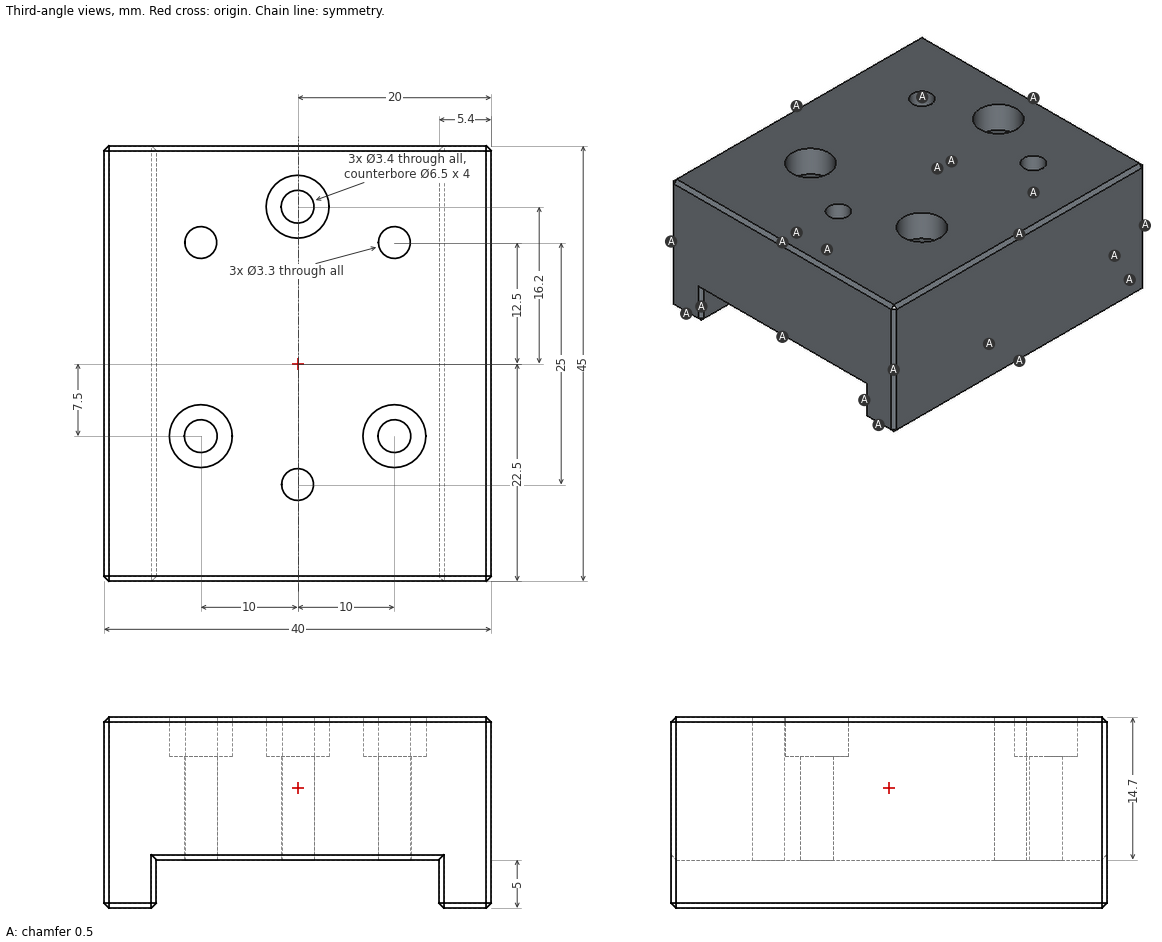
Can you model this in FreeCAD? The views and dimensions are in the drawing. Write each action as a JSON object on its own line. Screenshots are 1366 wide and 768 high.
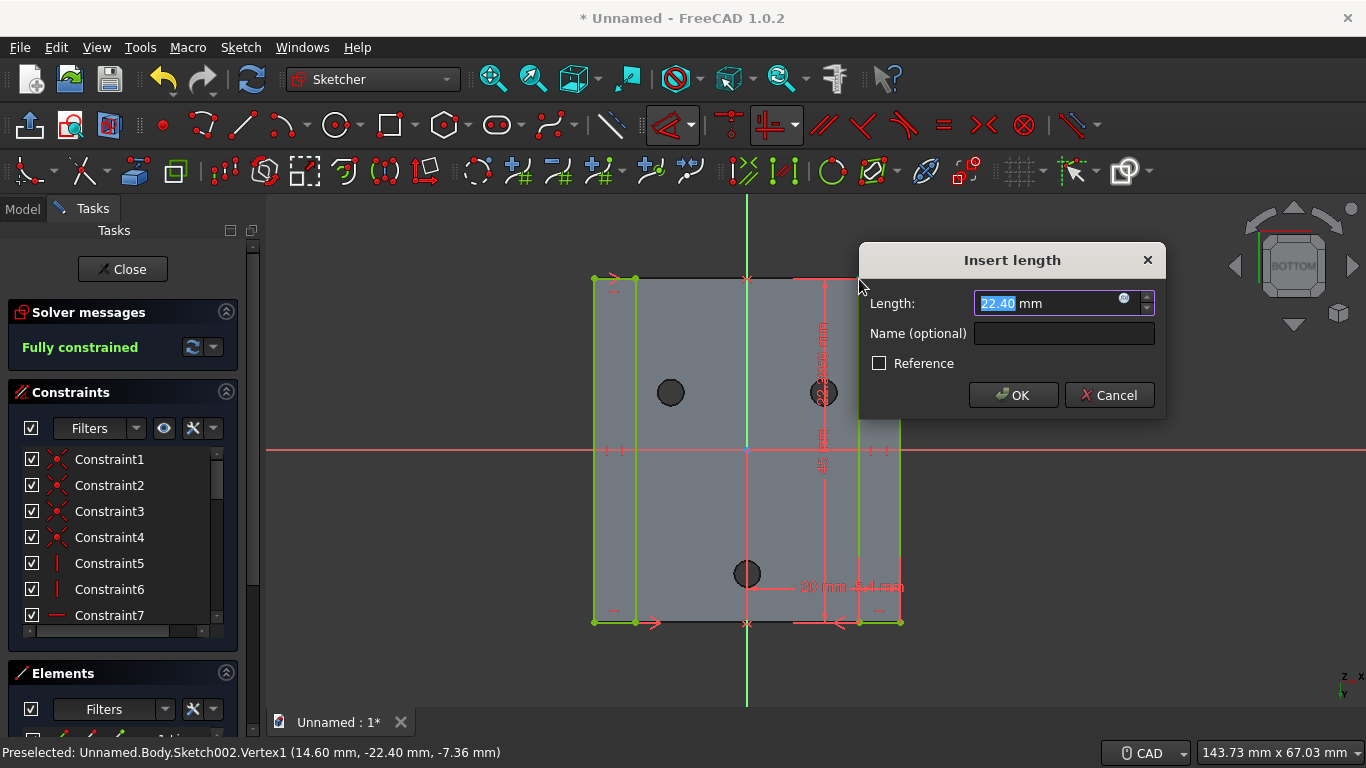
{"action": "type", "text": "22.5"}
{"action": "key", "text": "Return"}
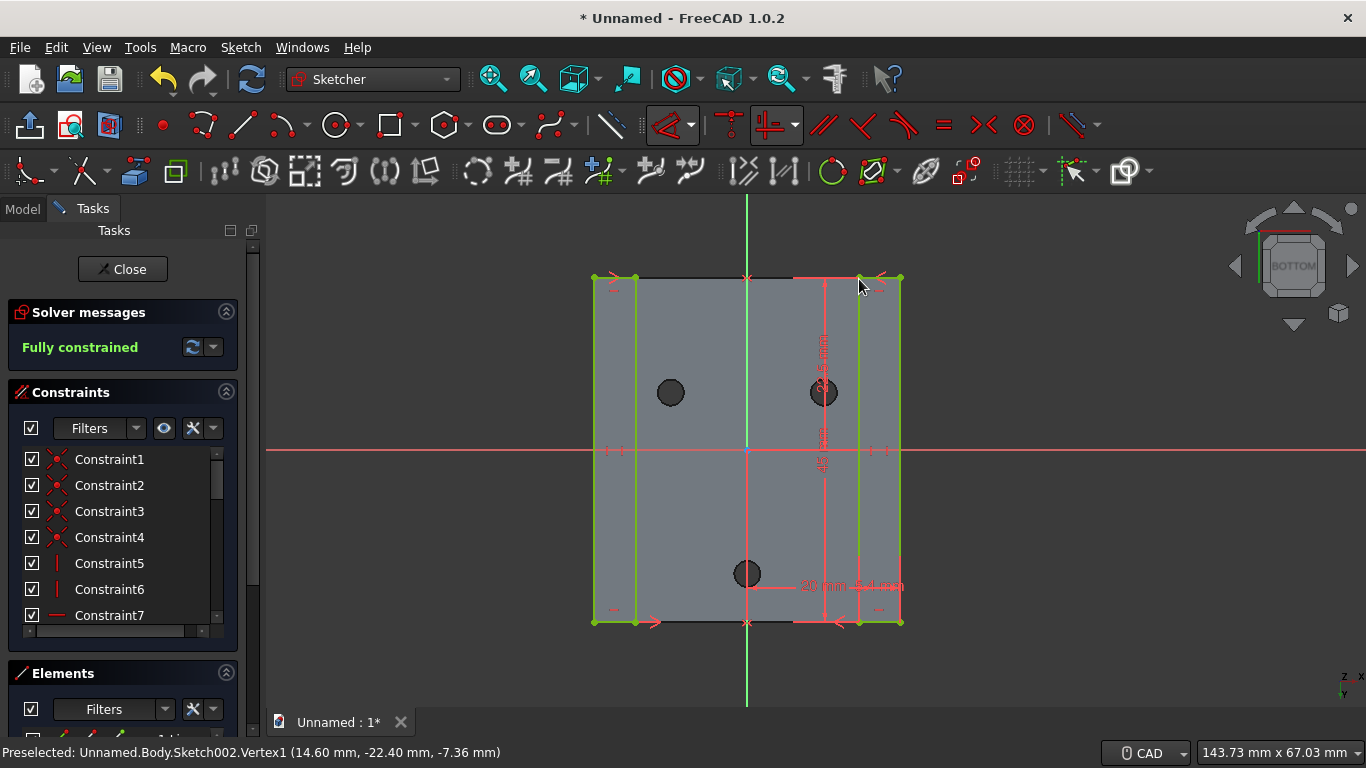
{"action": "left_click", "coordinate": [123, 269]}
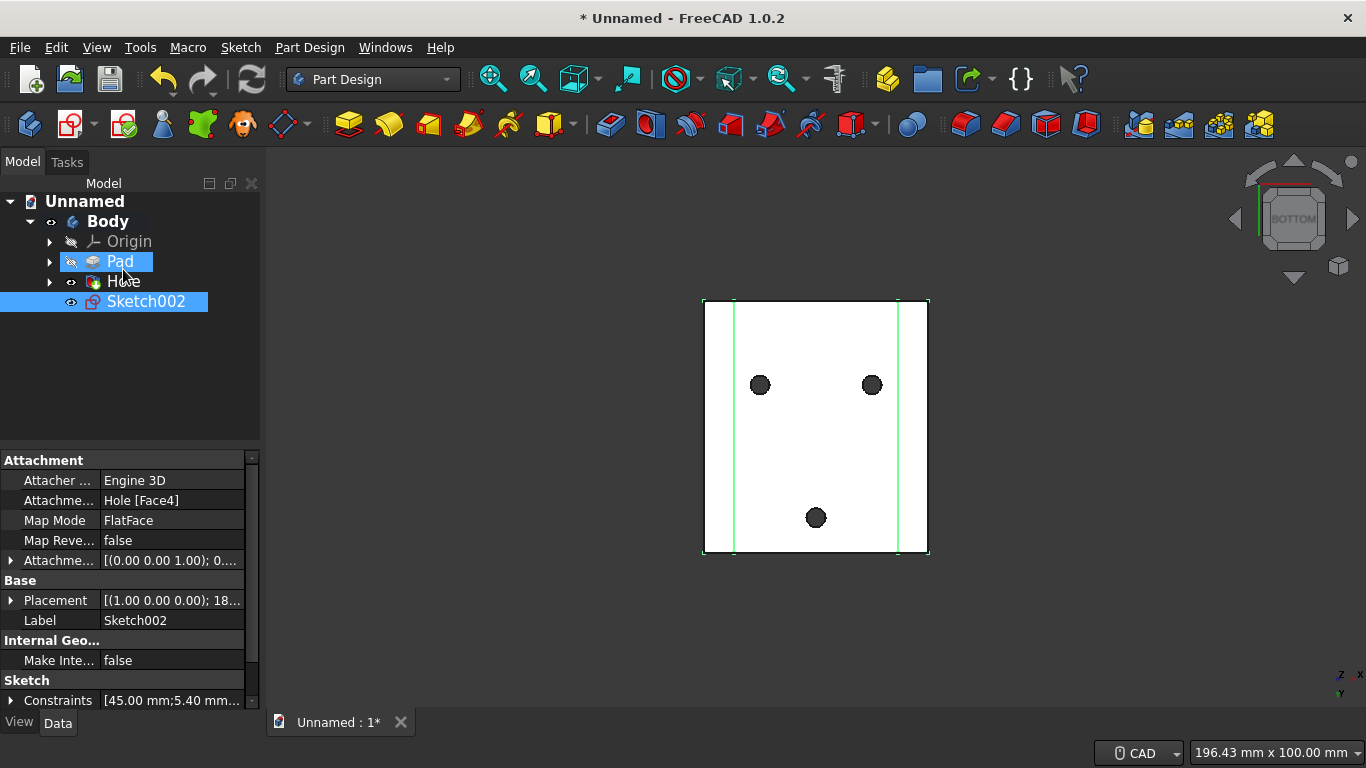
{"action": "left_click", "coordinate": [350, 124]}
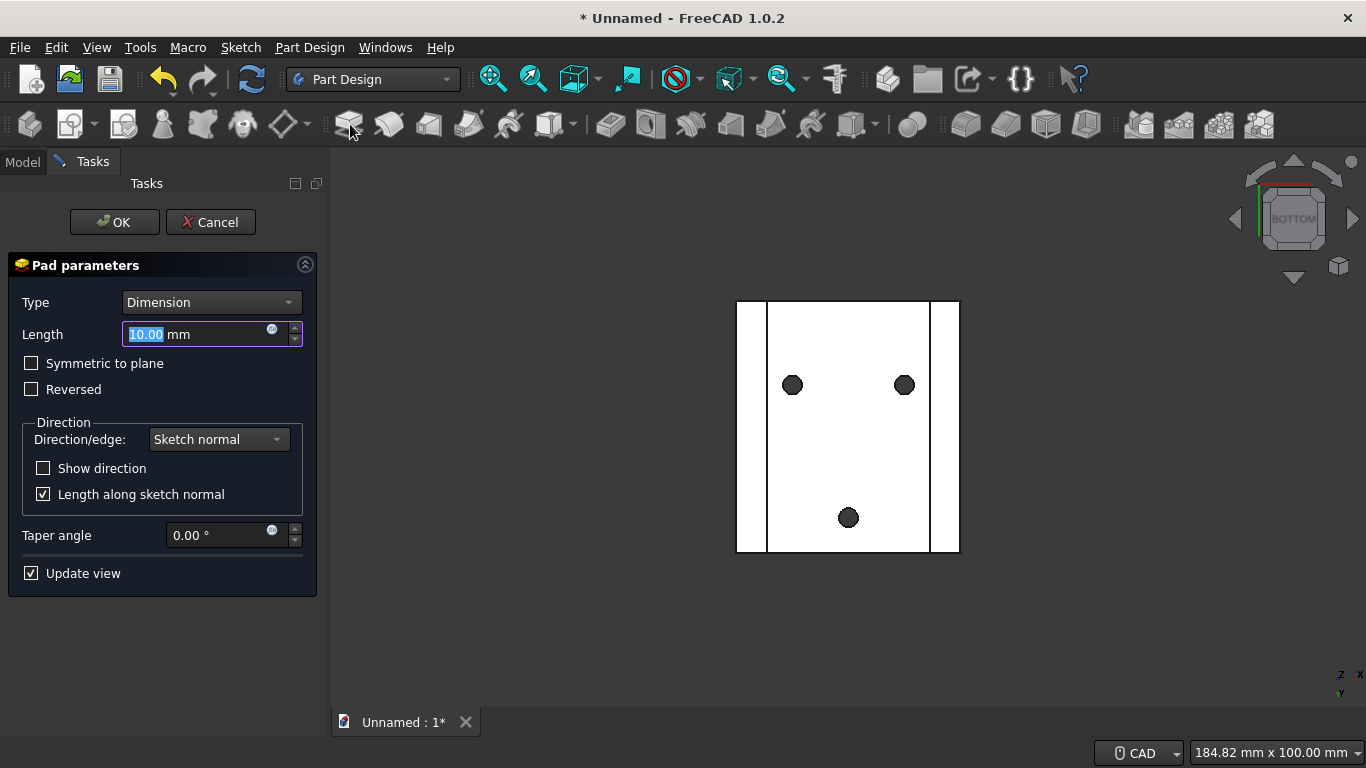
{"action": "type", "text": "5"}
{"action": "key", "text": "Tab"}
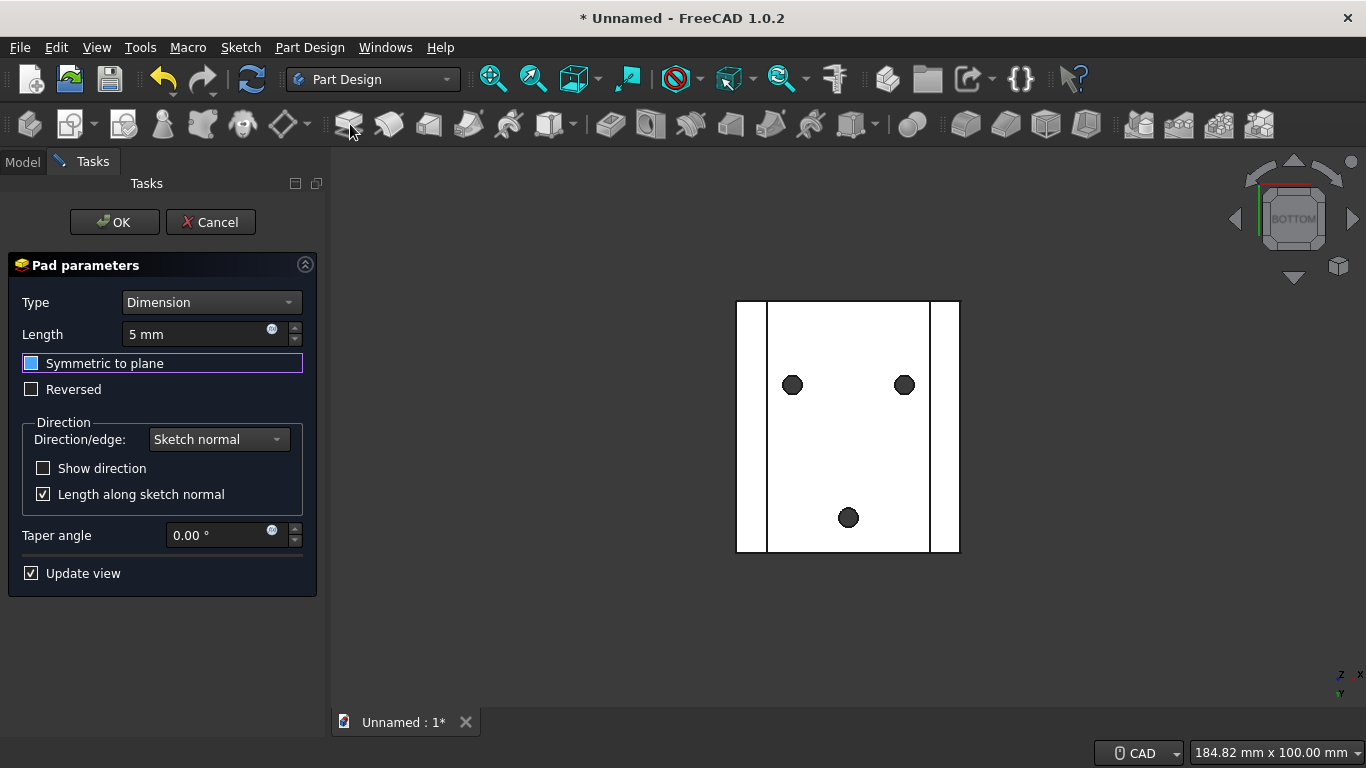
{"action": "left_click", "coordinate": [115, 222]}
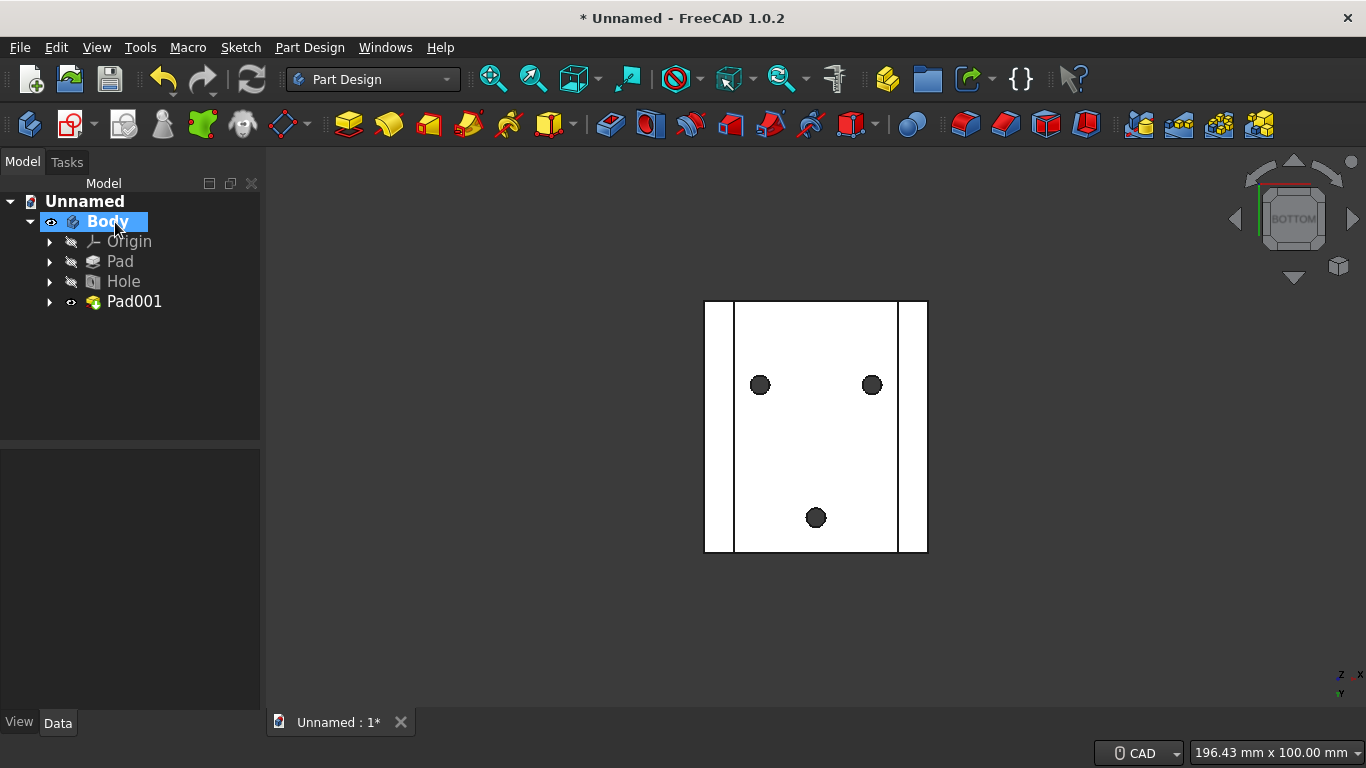
{"action": "key", "text": "0"}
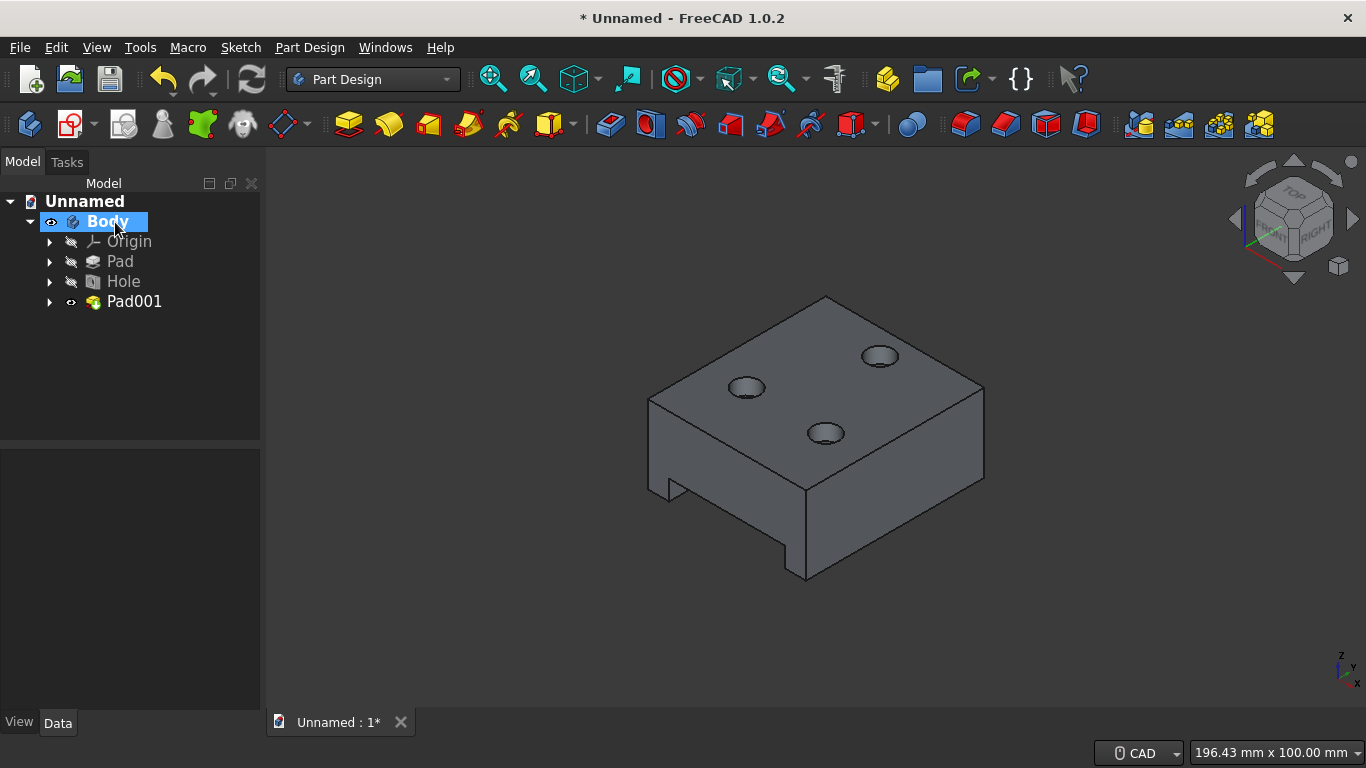
{"action": "left_click", "coordinate": [816, 392]}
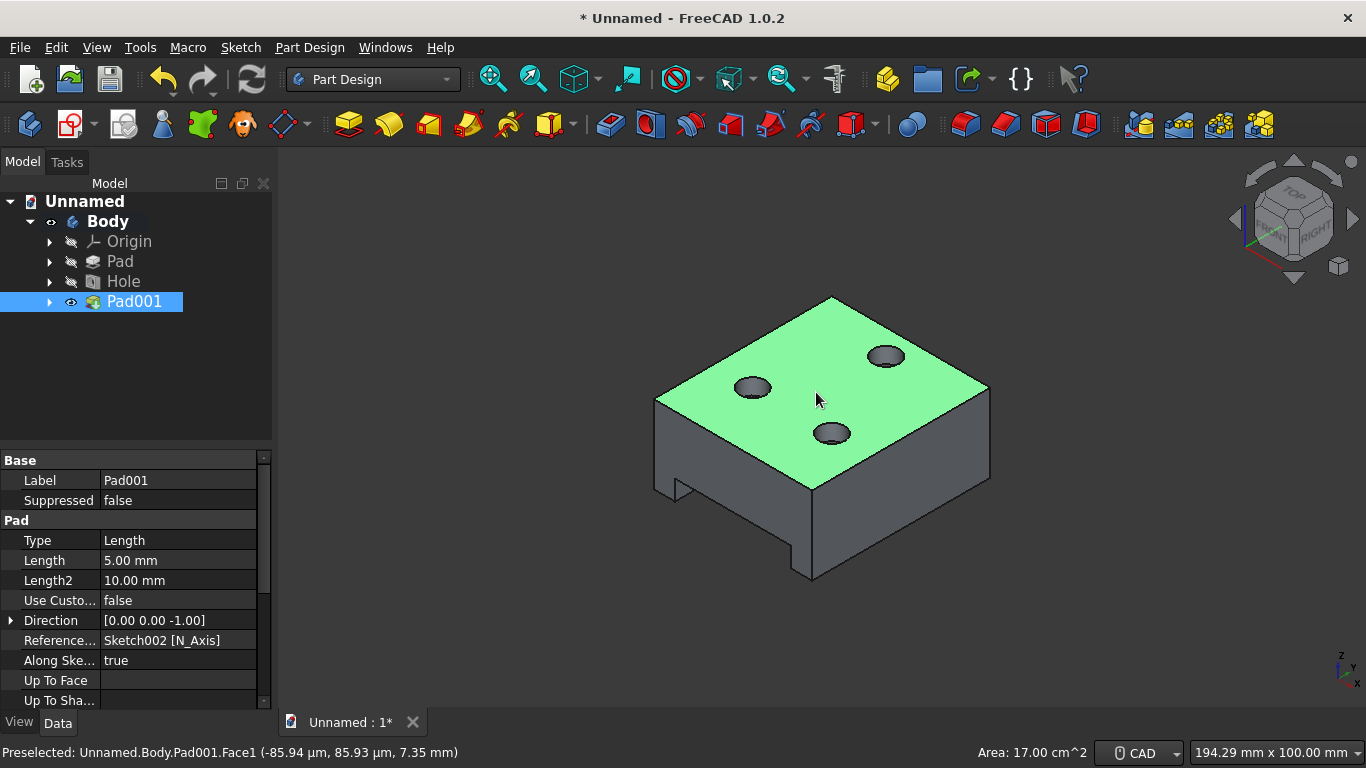
{"action": "left_click", "coordinate": [70, 124]}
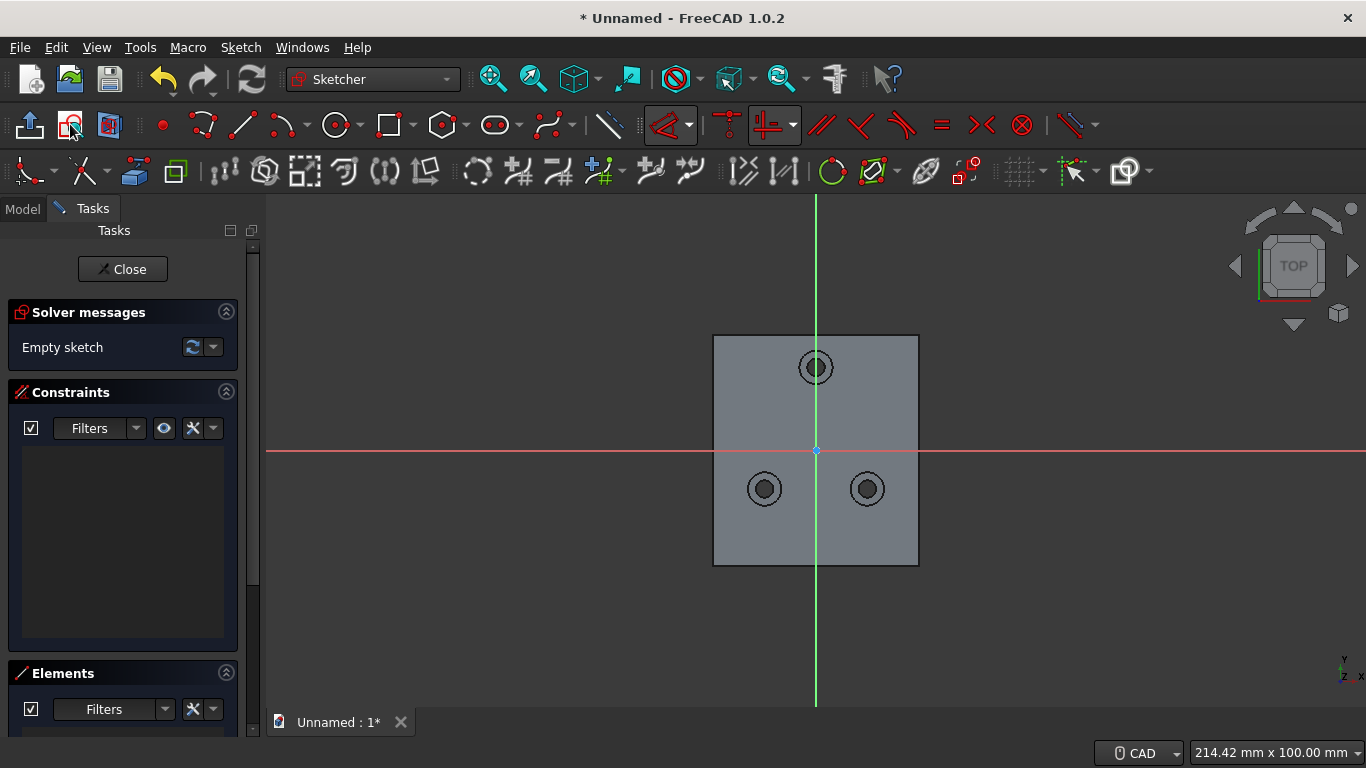
{"action": "scroll", "coordinate": [872, 450], "scroll_direction": "up", "scroll_amount": 4}